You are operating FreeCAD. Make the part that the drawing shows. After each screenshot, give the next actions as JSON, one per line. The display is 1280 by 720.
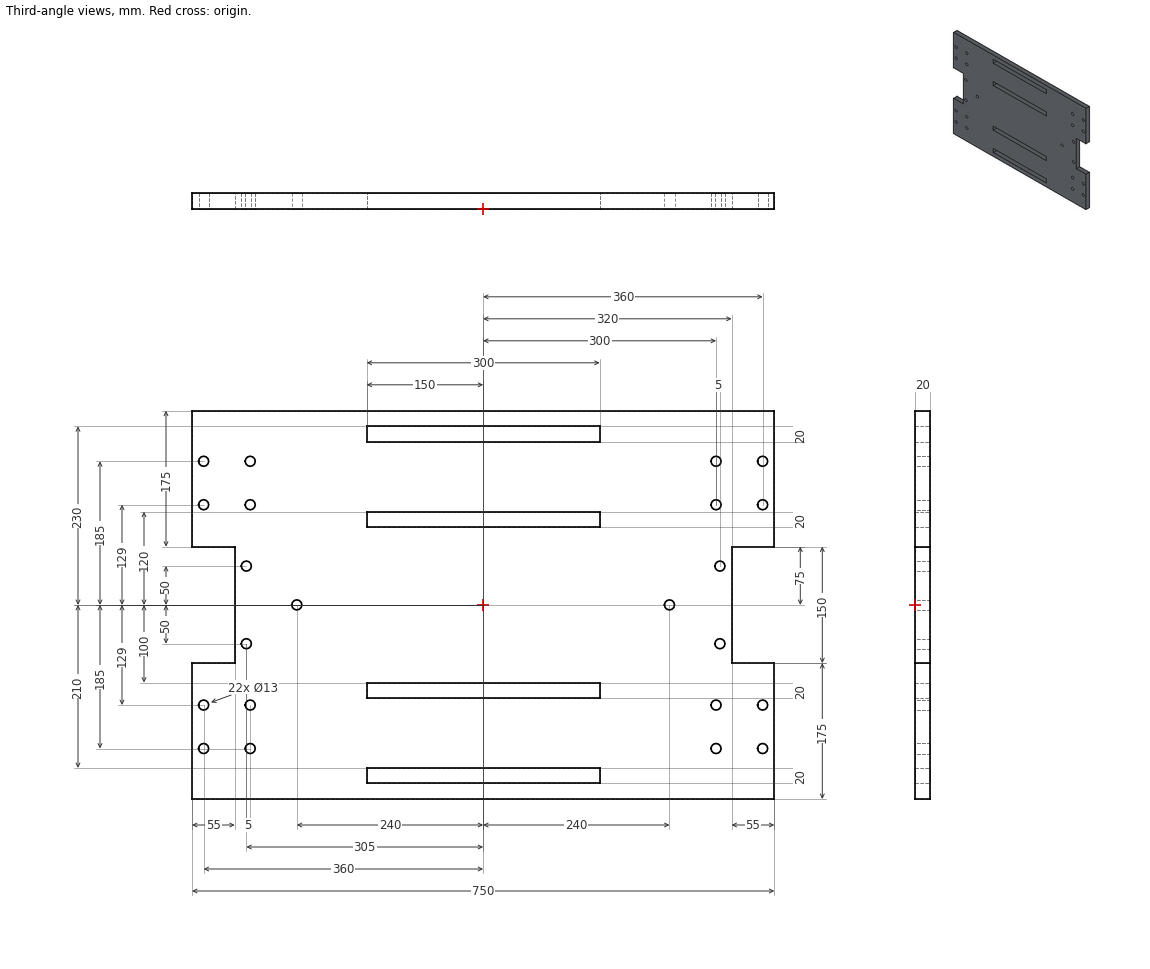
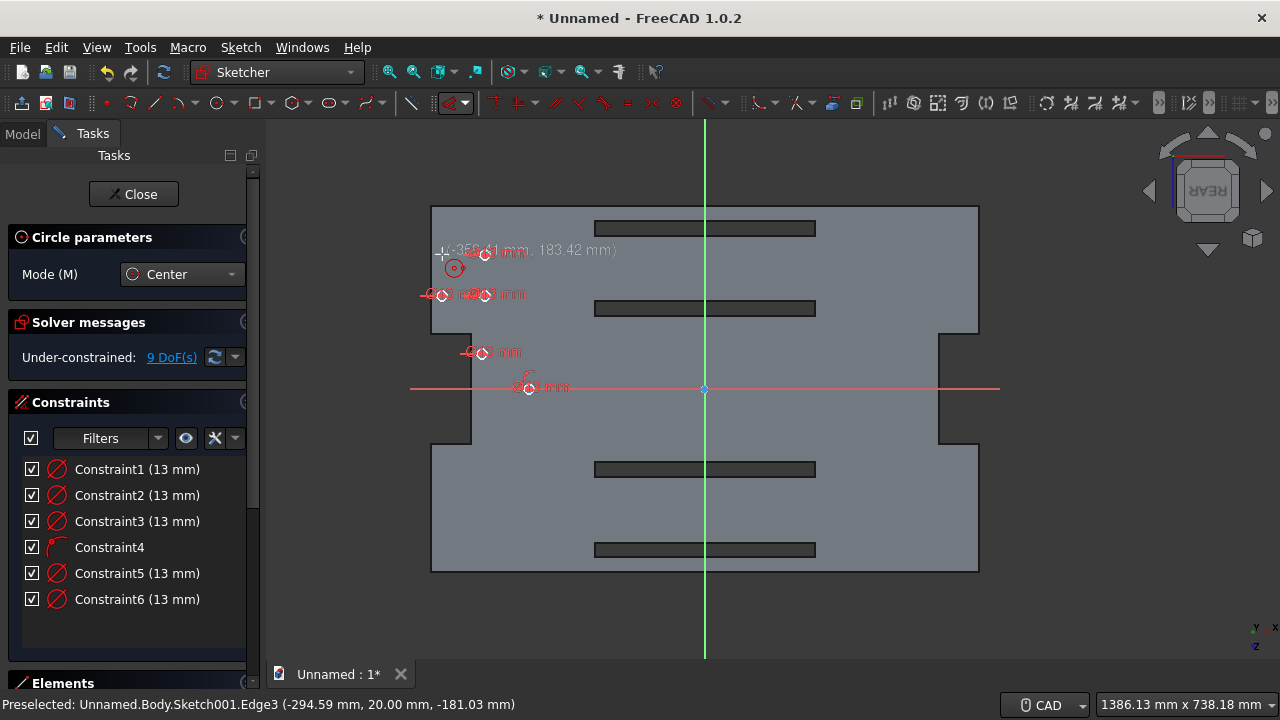
{"action": "left_click", "coordinate": [442, 254]}
{"action": "mouse_move", "coordinate": [445, 250]}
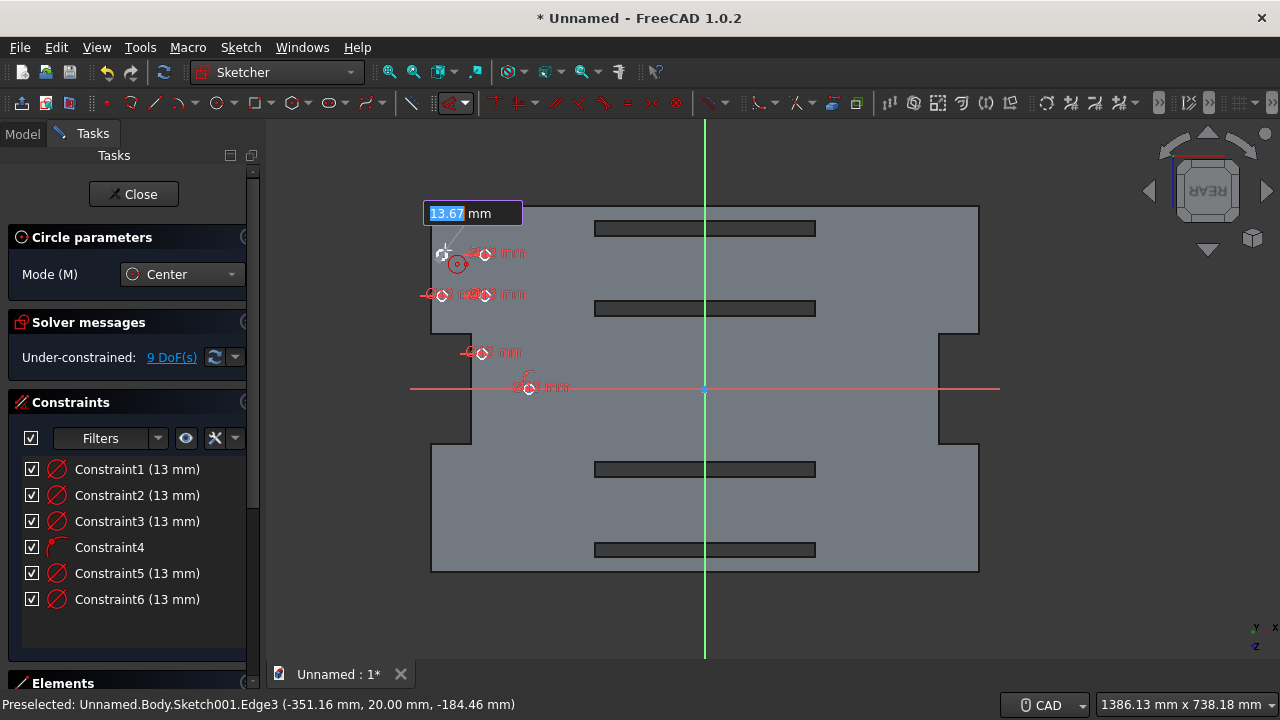
{"action": "type", "text": "13"}
{"action": "key", "text": "Return"}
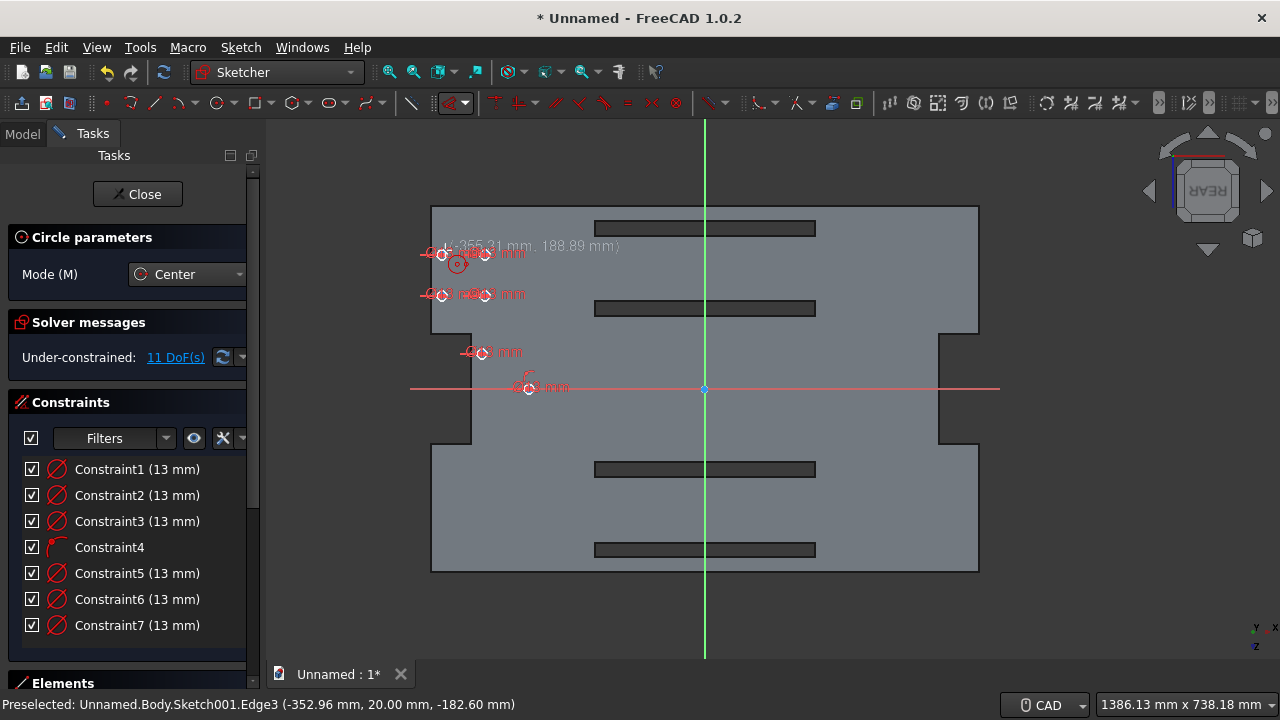
{"action": "scroll", "coordinate": [442, 484], "scroll_direction": "up", "scroll_amount": 8}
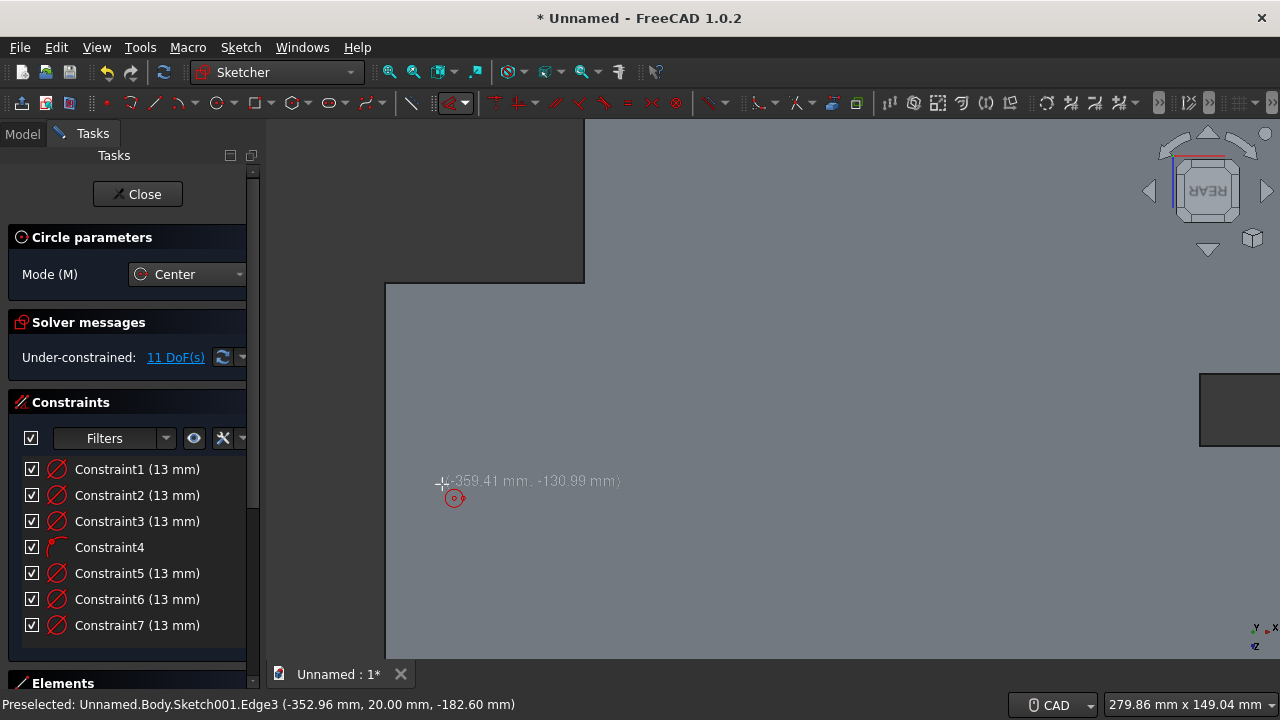
{"action": "scroll", "coordinate": [442, 484], "scroll_direction": "down", "scroll_amount": 8}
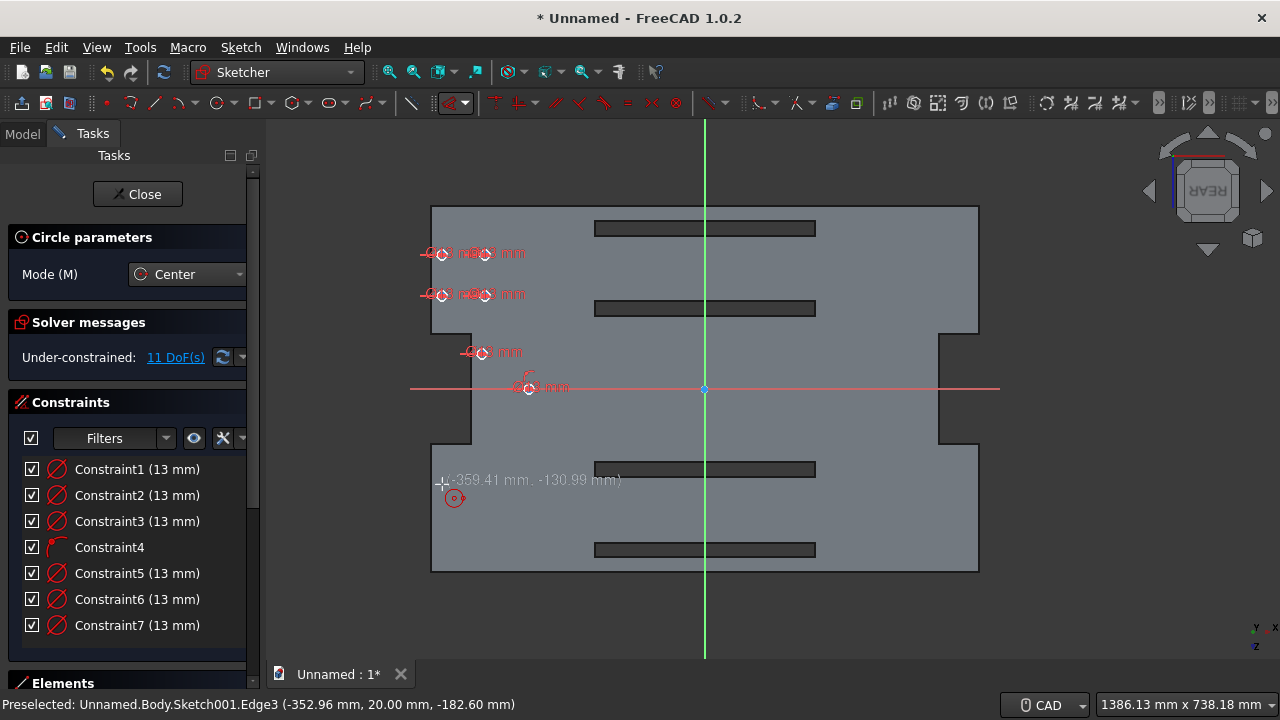
{"action": "left_click", "coordinate": [442, 484]}
{"action": "mouse_move", "coordinate": [445, 480]}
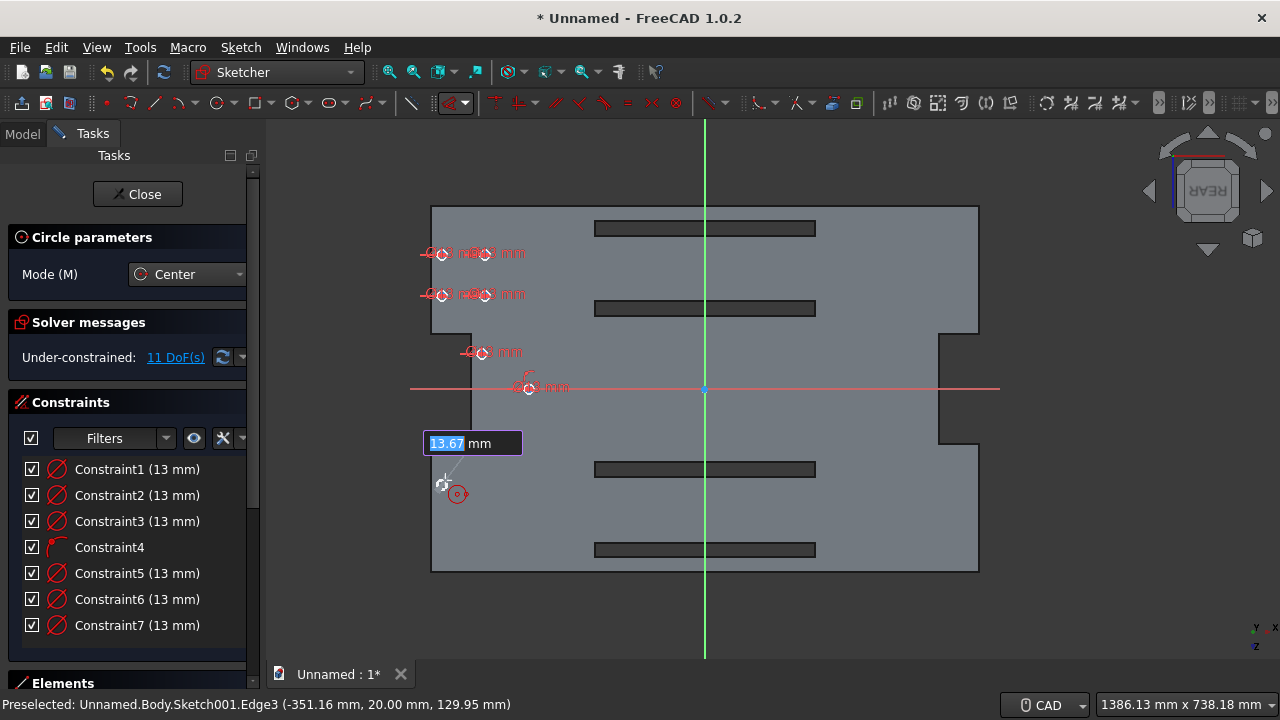
{"action": "type", "text": "13"}
{"action": "key", "text": "Return"}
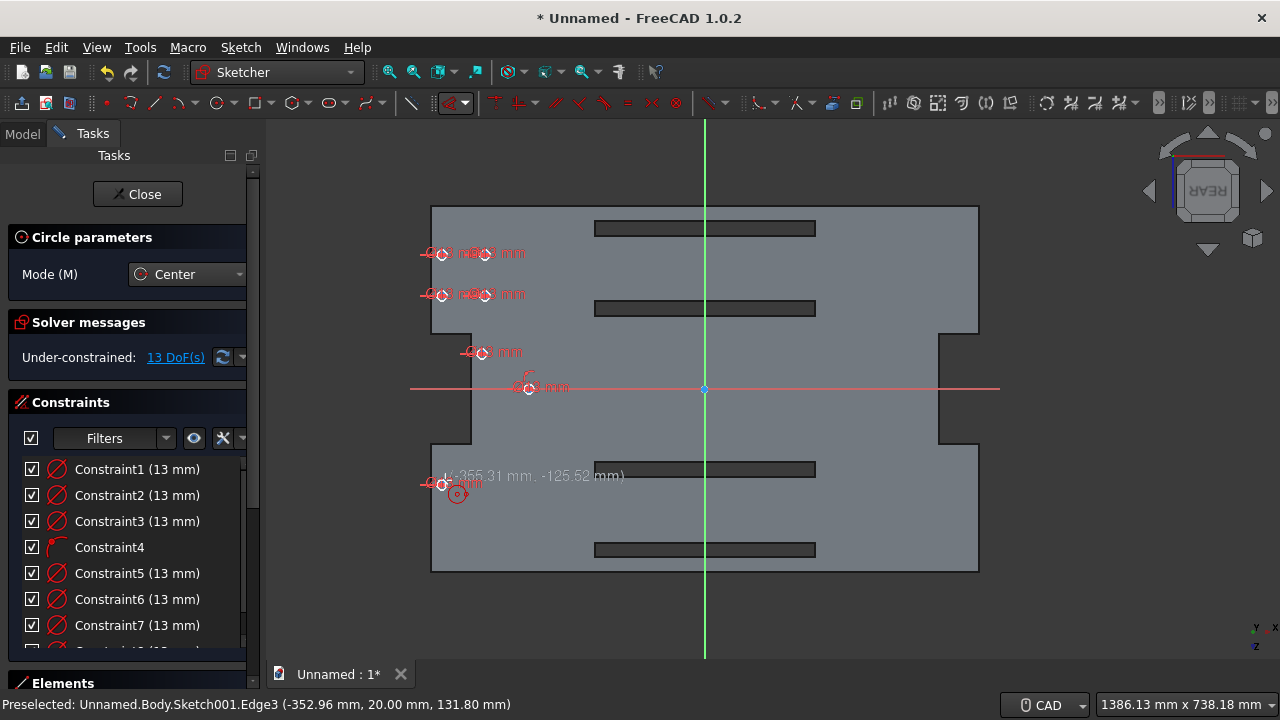
{"action": "scroll", "coordinate": [442, 525], "scroll_direction": "up", "scroll_amount": 8}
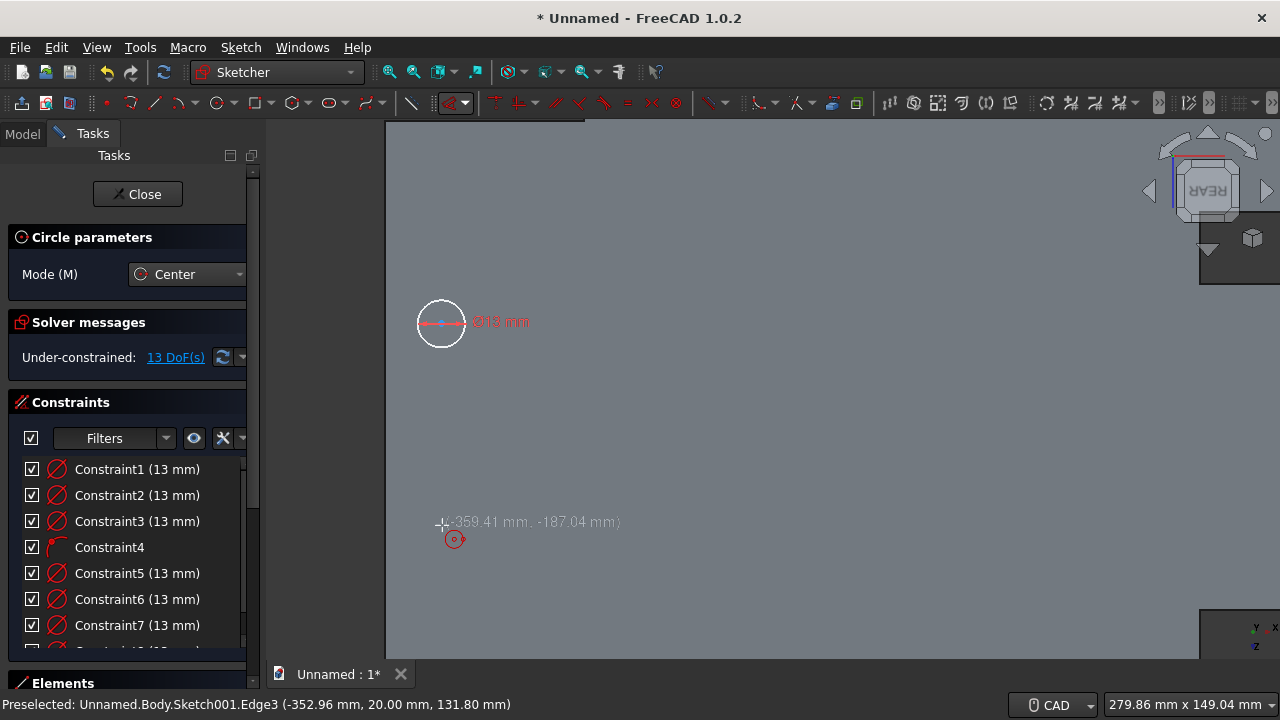
{"action": "scroll", "coordinate": [442, 526], "scroll_direction": "down", "scroll_amount": 8}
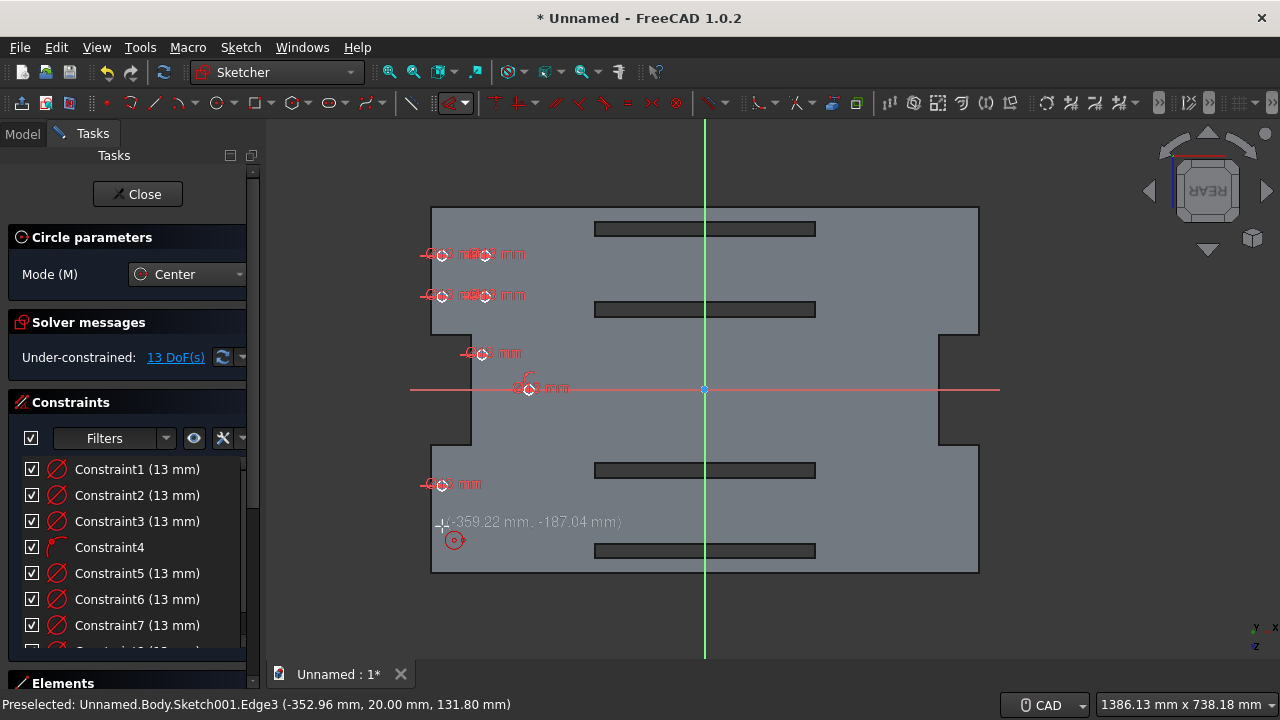
{"action": "left_click", "coordinate": [442, 525]}
{"action": "mouse_move", "coordinate": [445, 522]}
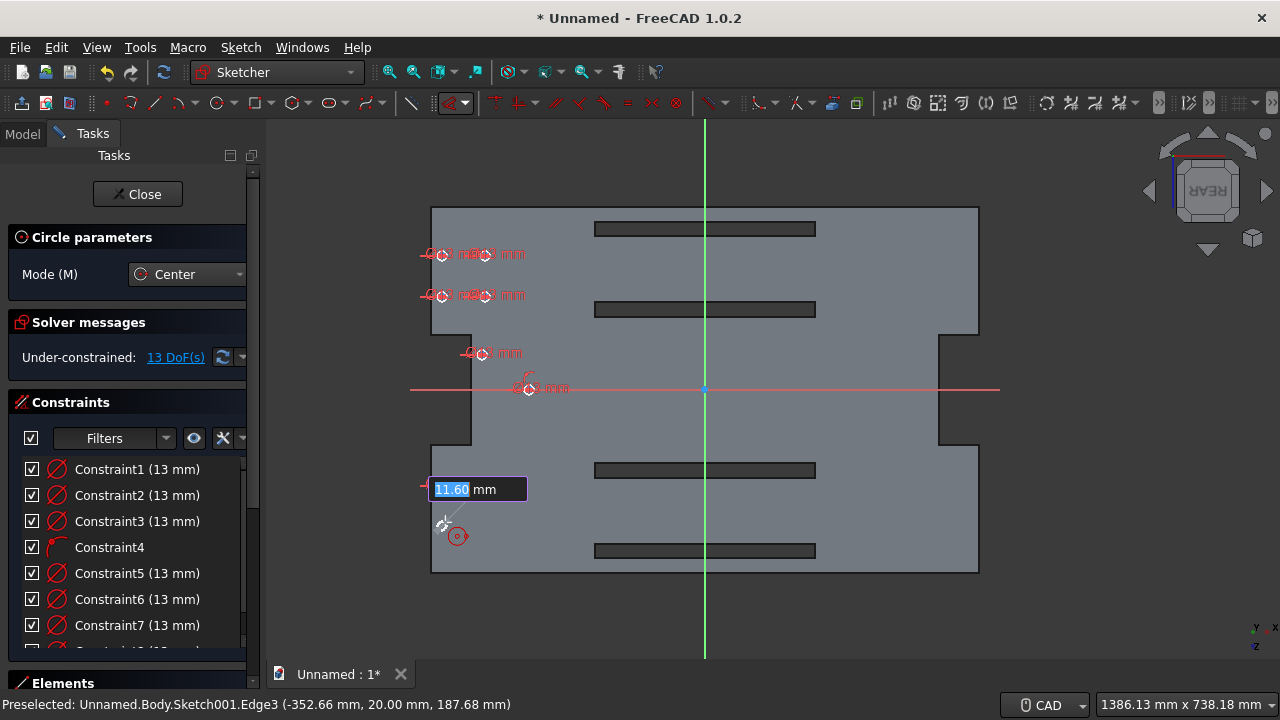
{"action": "type", "text": "13"}
{"action": "key", "text": "Return"}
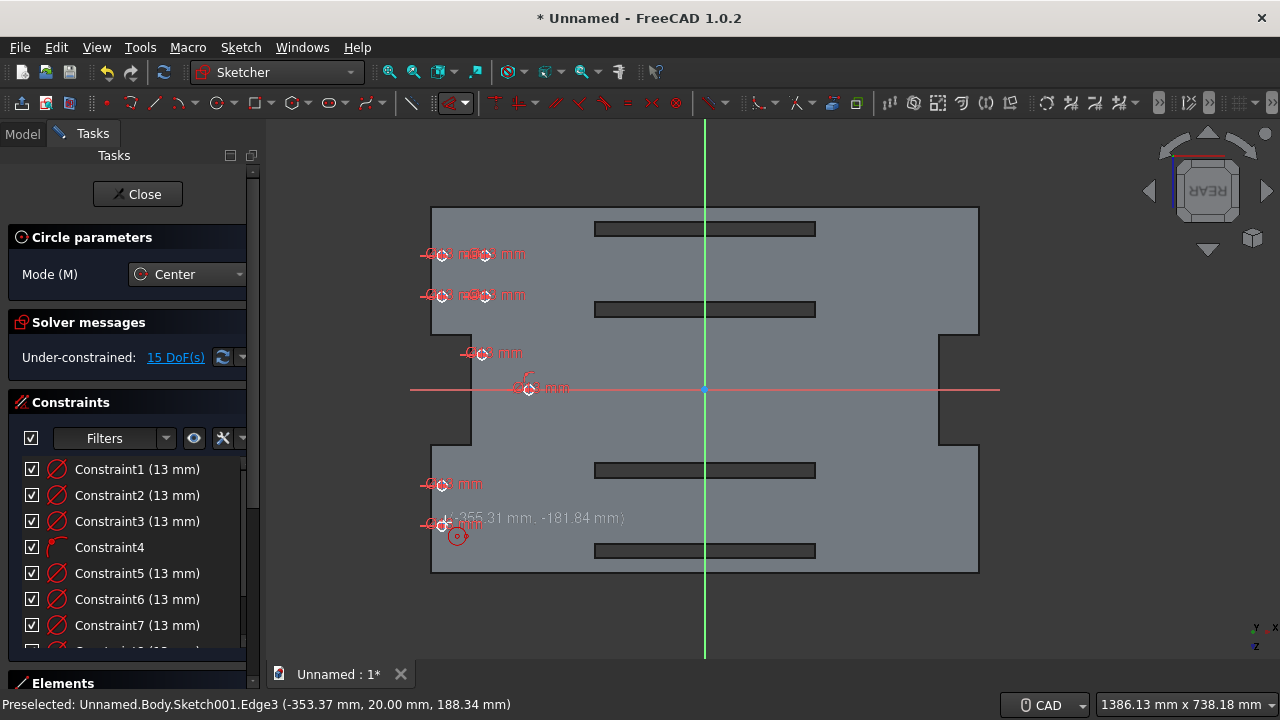
{"action": "scroll", "coordinate": [485, 484], "scroll_direction": "up", "scroll_amount": 8}